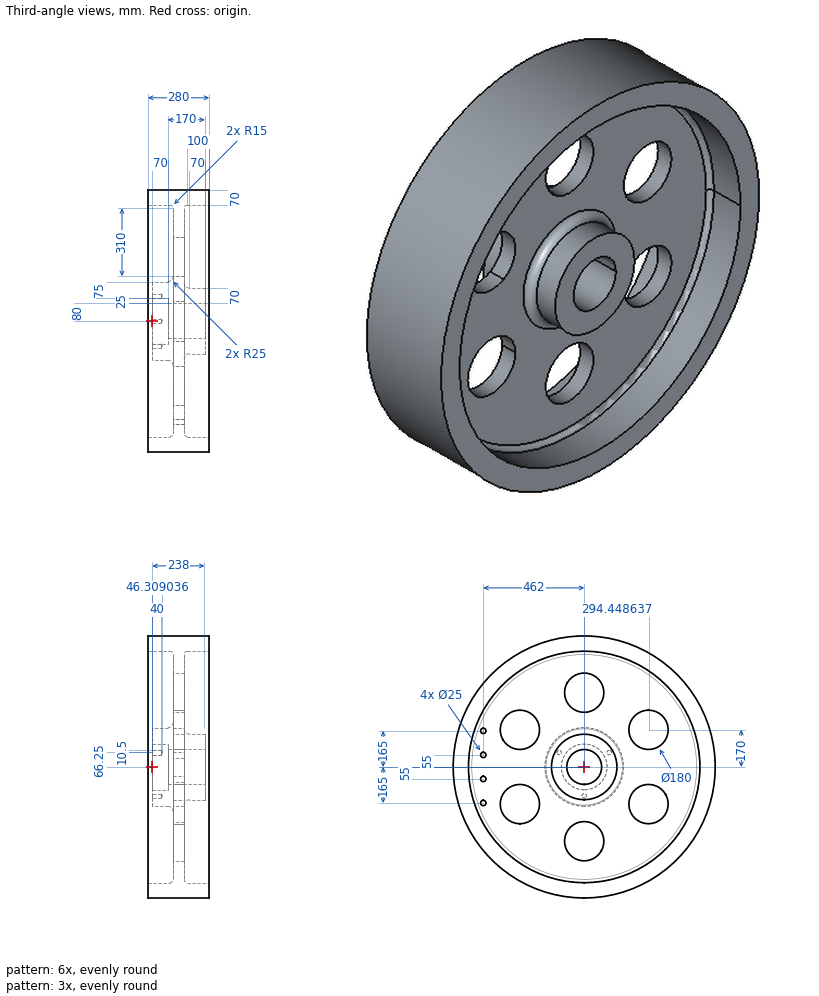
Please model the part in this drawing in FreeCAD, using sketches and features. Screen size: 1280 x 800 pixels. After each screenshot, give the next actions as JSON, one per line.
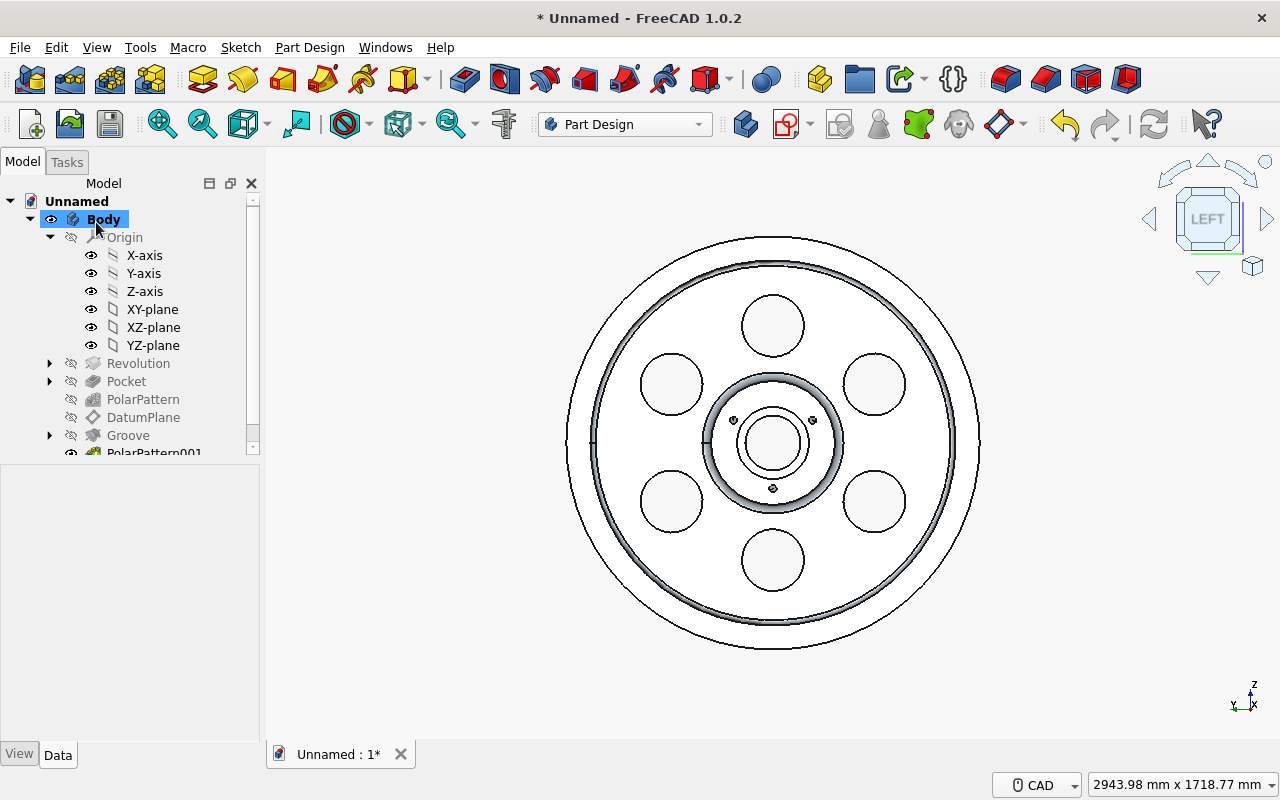
{"action": "left_click", "coordinate": [786, 124]}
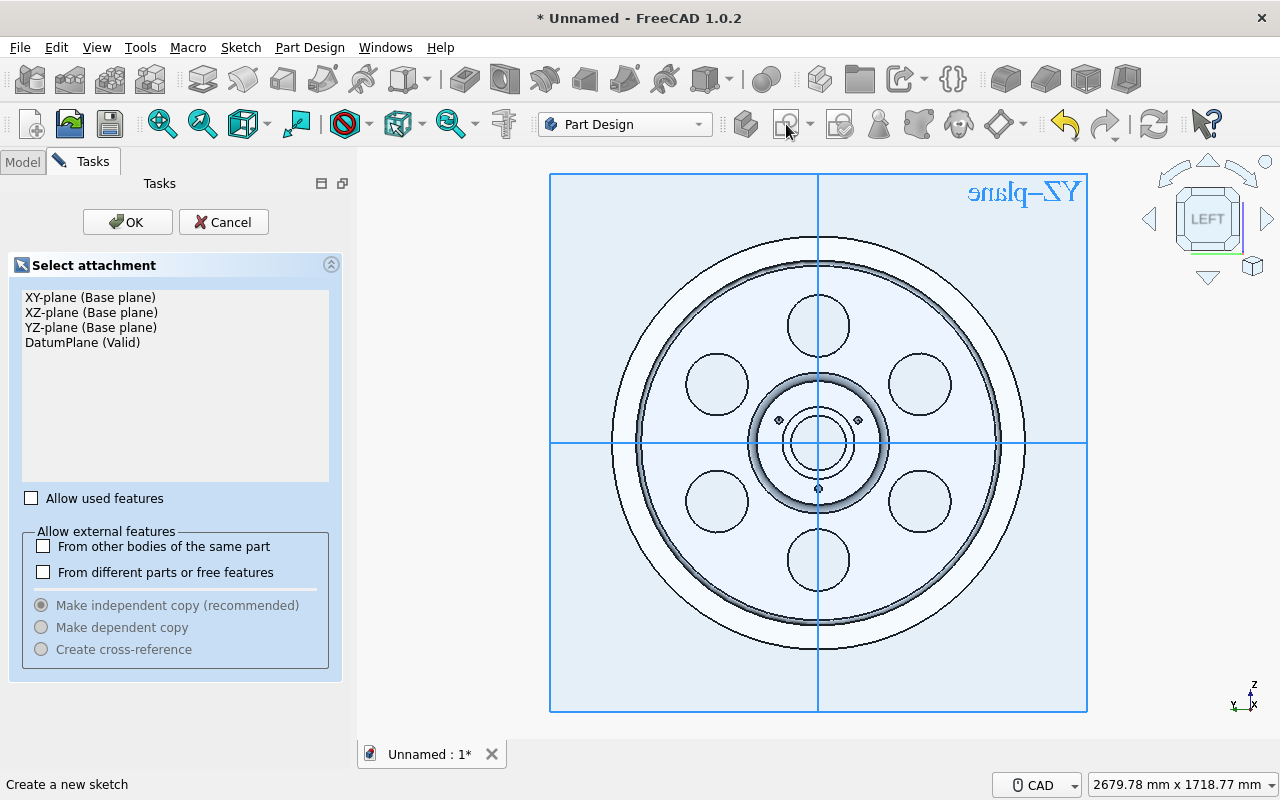
{"action": "left_click", "coordinate": [82, 328]}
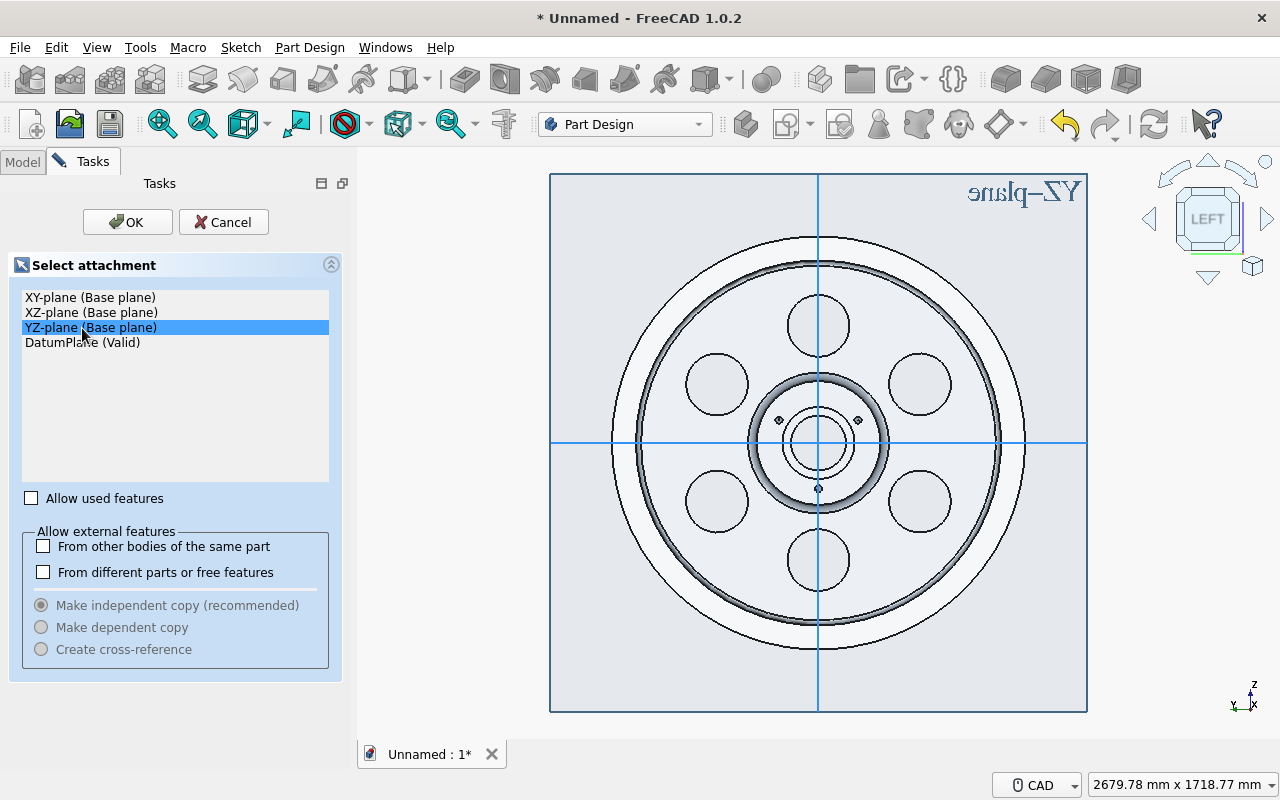
{"action": "left_click", "coordinate": [128, 222]}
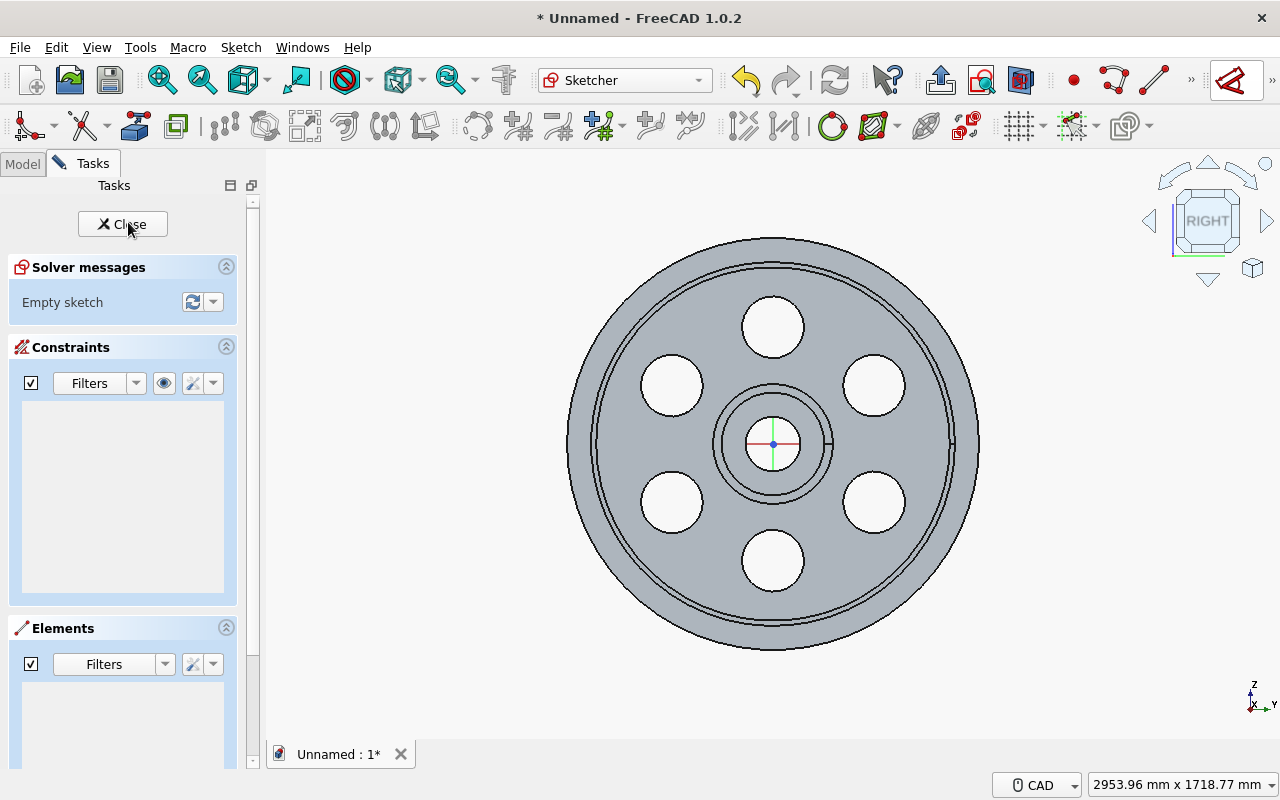
{"action": "left_click", "coordinate": [1022, 80]}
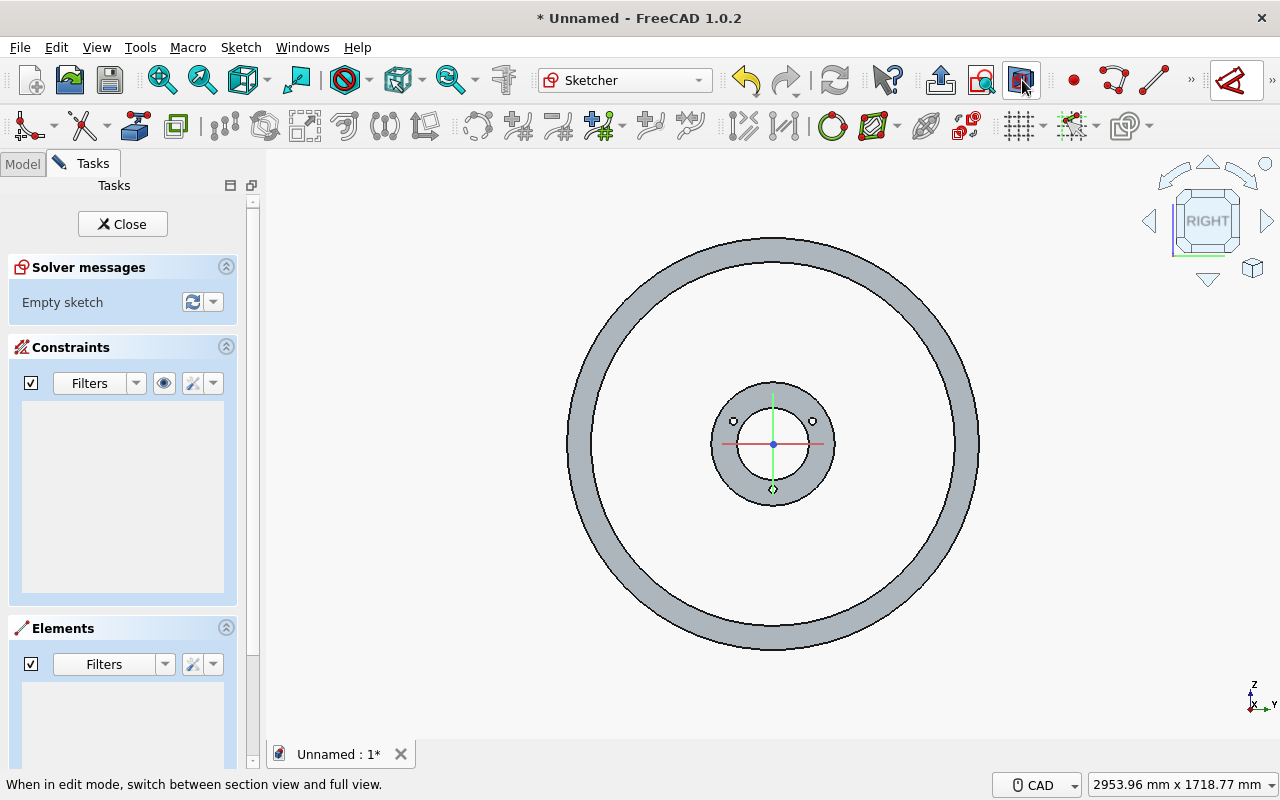
{"action": "scroll", "coordinate": [686, 444], "scroll_direction": "up", "scroll_amount": 6}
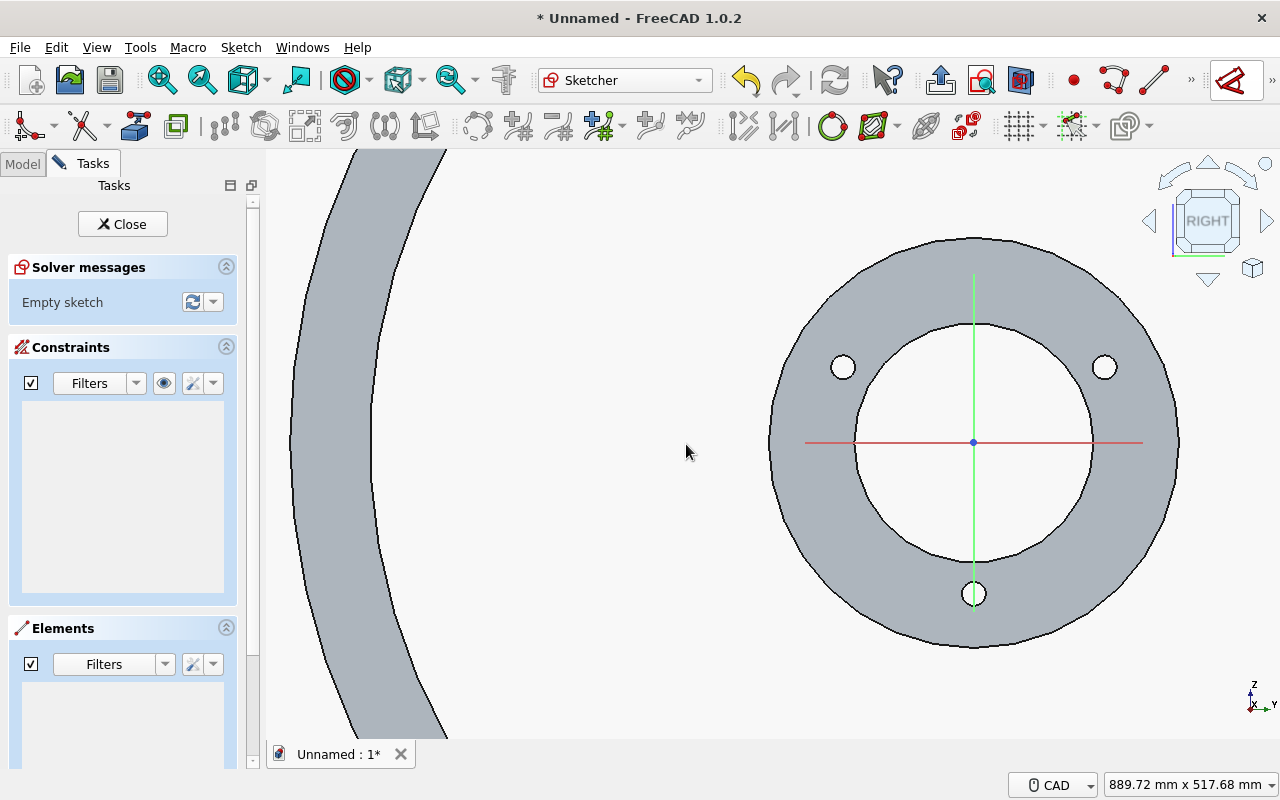
{"action": "key", "text": "g c"}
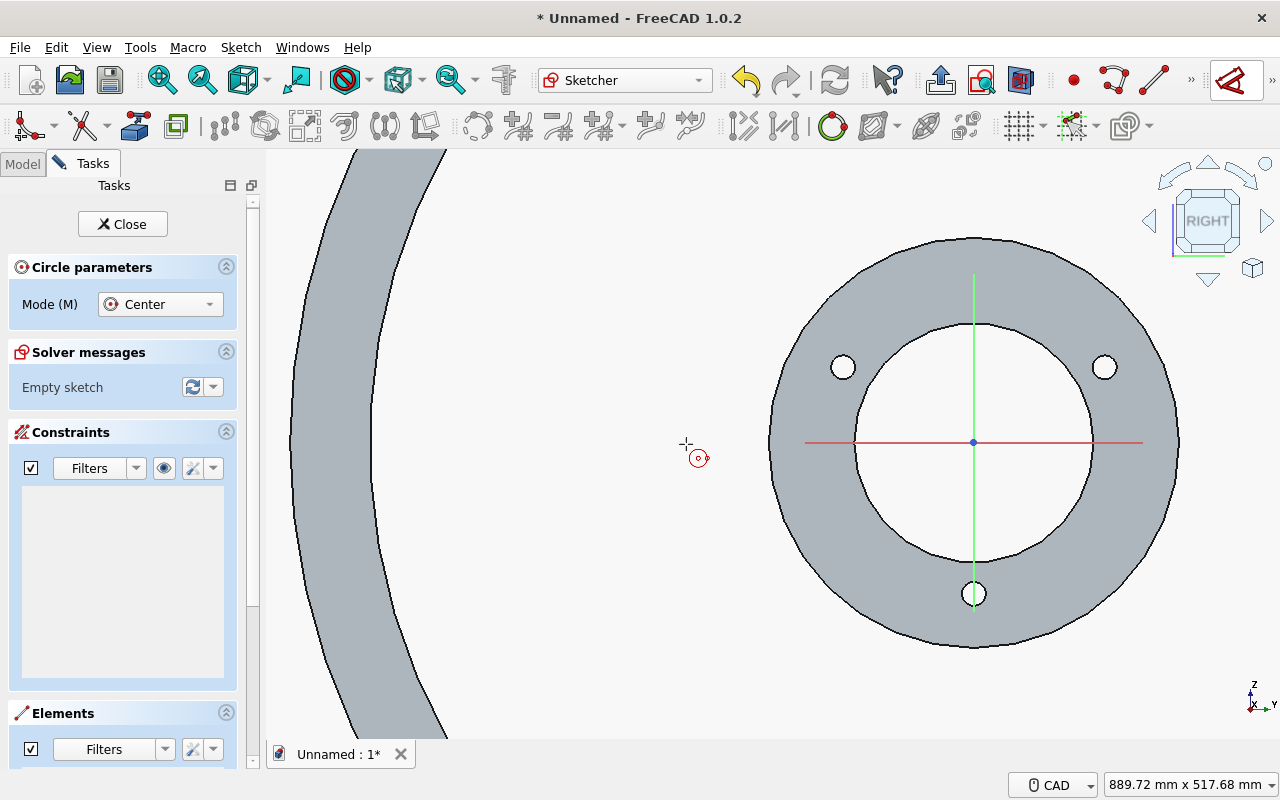
{"action": "scroll", "coordinate": [447, 380], "scroll_direction": "up", "scroll_amount": 3}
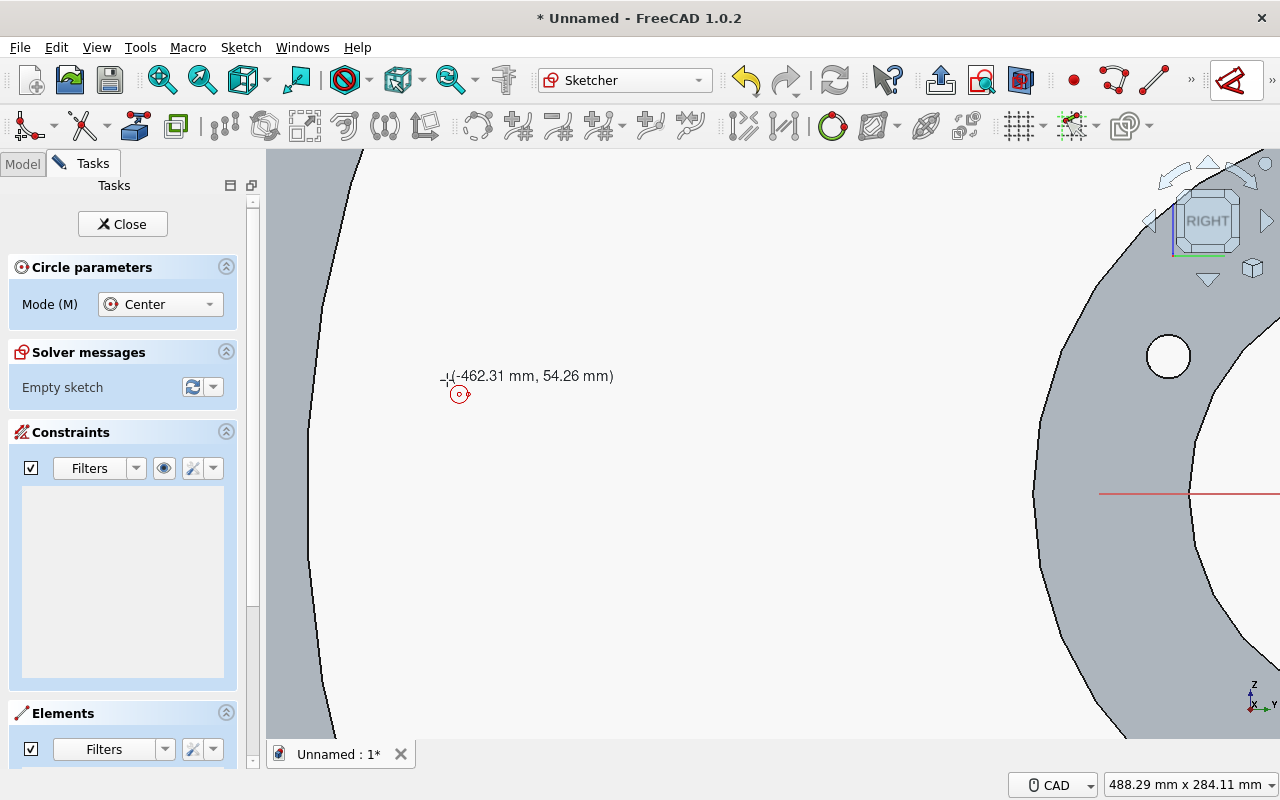
{"action": "left_click", "coordinate": [447, 380]}
{"action": "left_click", "coordinate": [466, 362]}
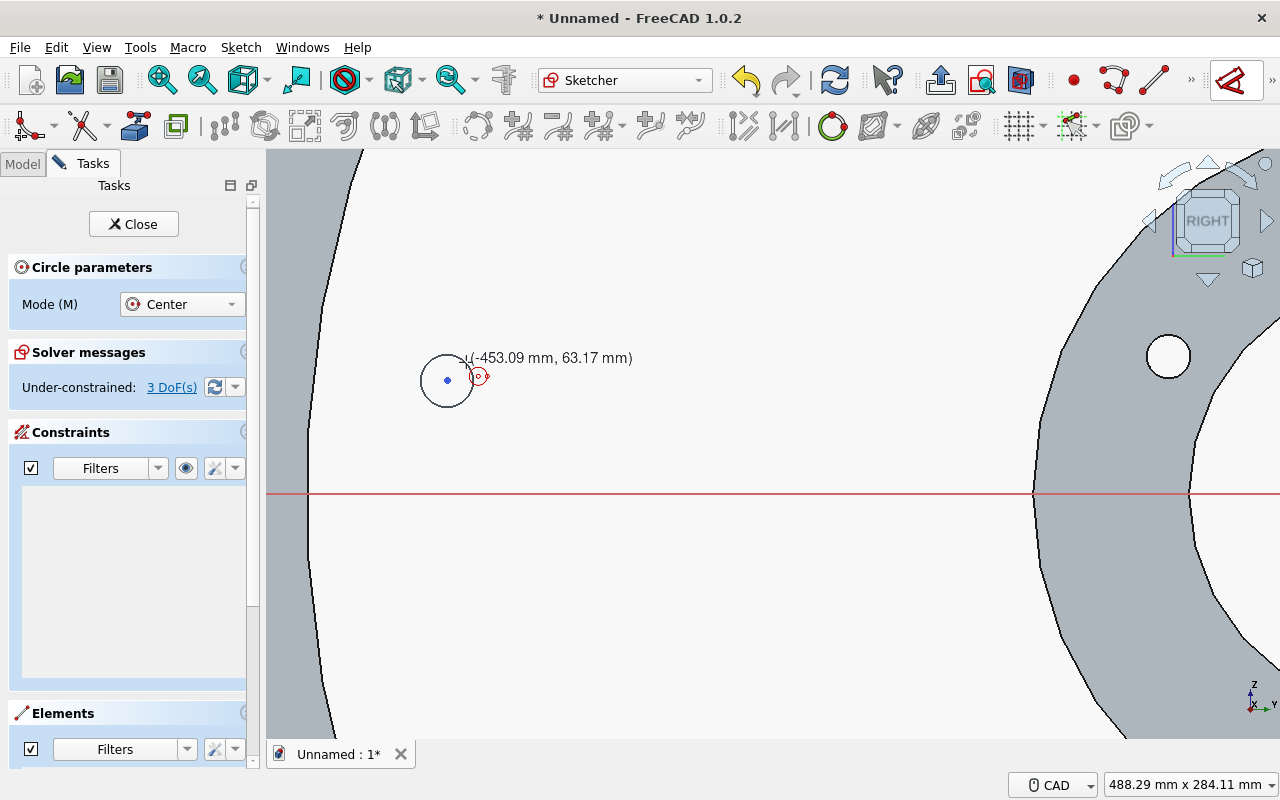
{"action": "scroll", "coordinate": [449, 383], "scroll_direction": "down", "scroll_amount": 3}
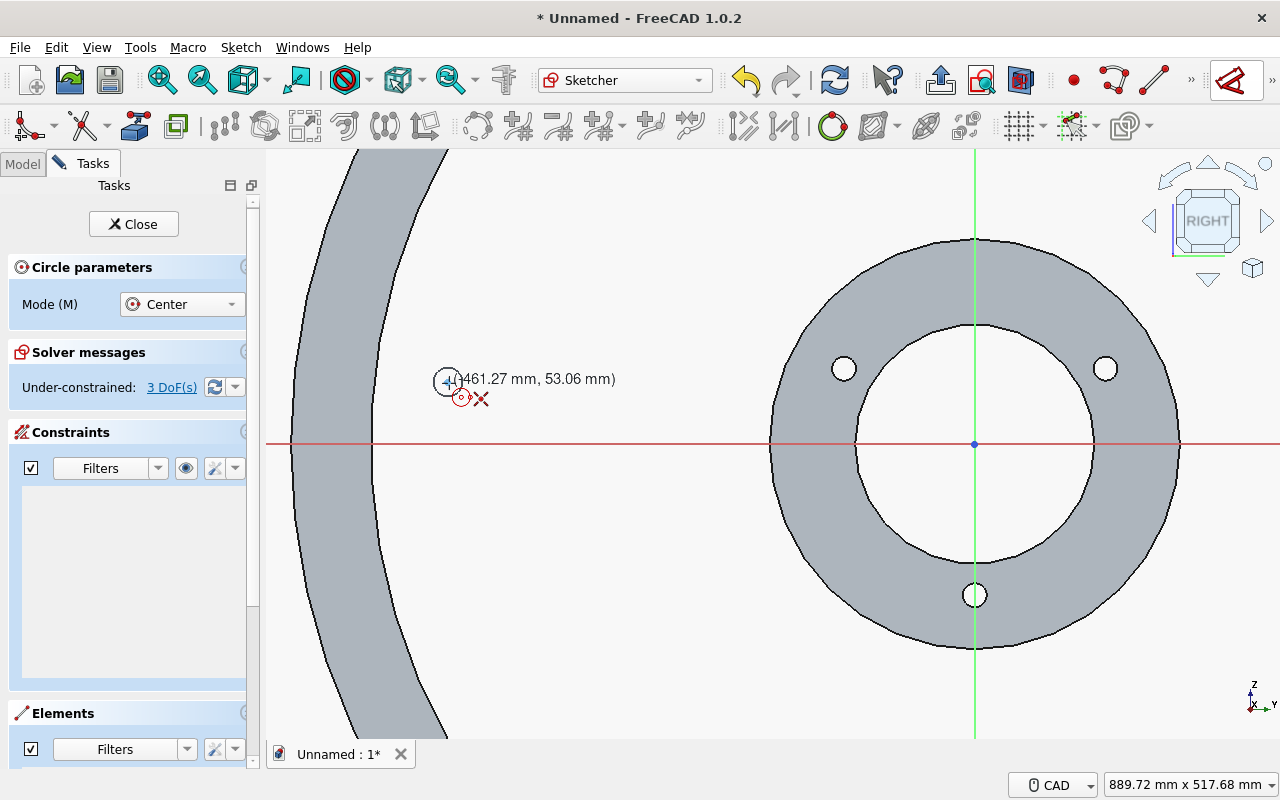
{"action": "scroll", "coordinate": [448, 256], "scroll_direction": "up", "scroll_amount": 3}